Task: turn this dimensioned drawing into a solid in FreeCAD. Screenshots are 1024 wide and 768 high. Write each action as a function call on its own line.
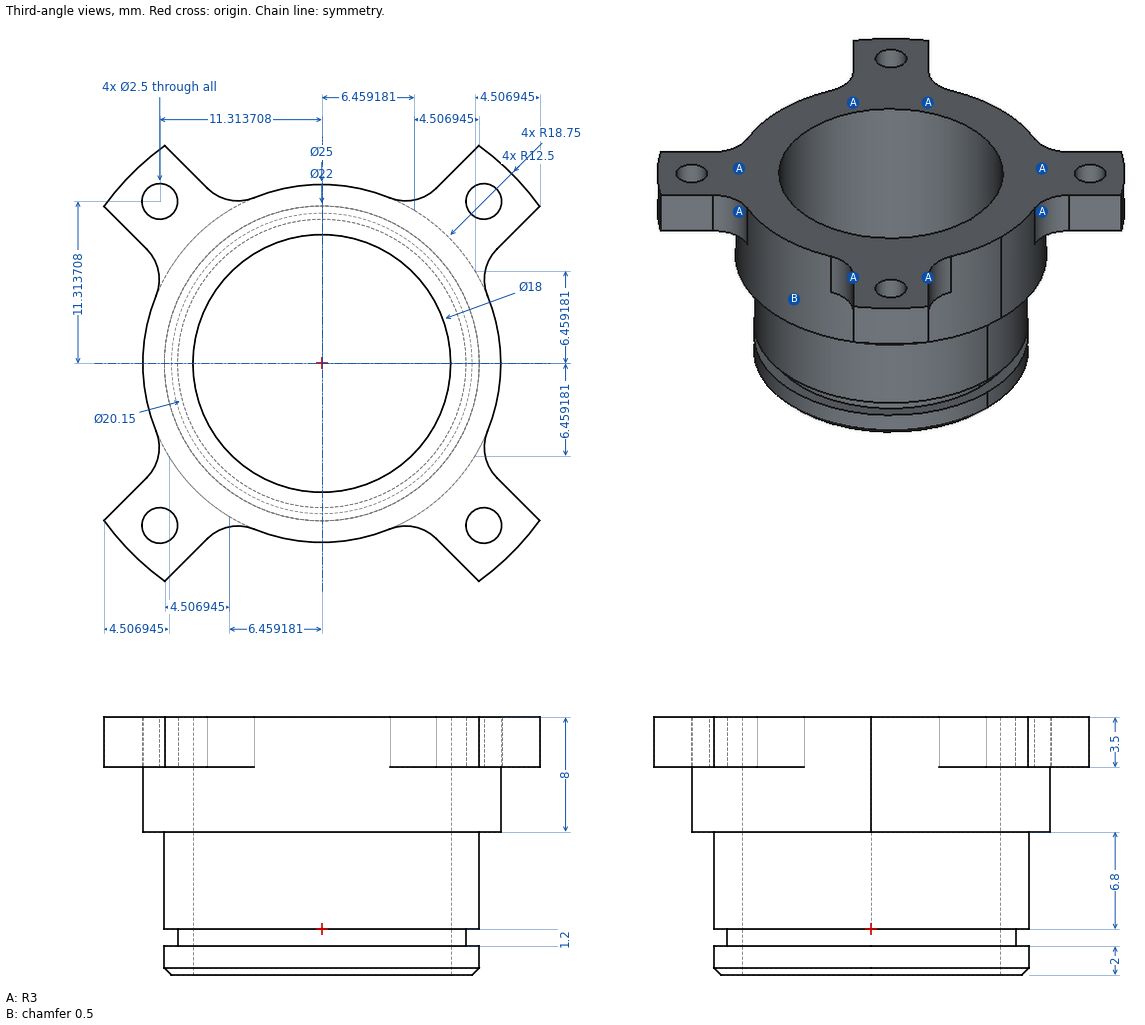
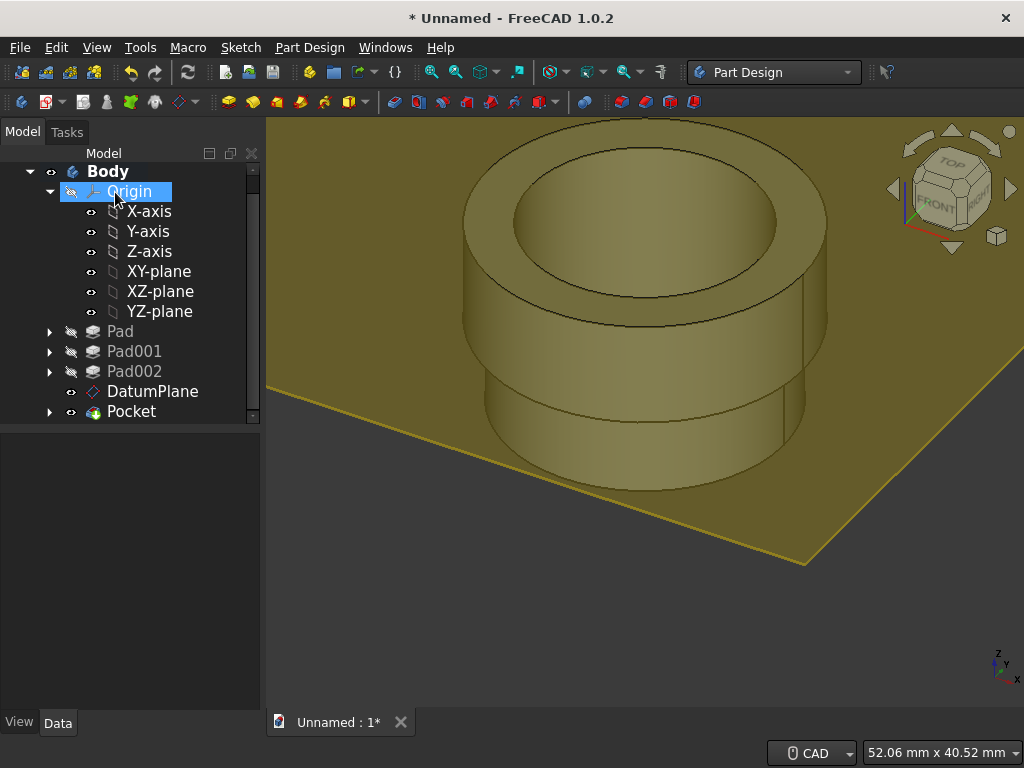
click(116, 392)
key(space)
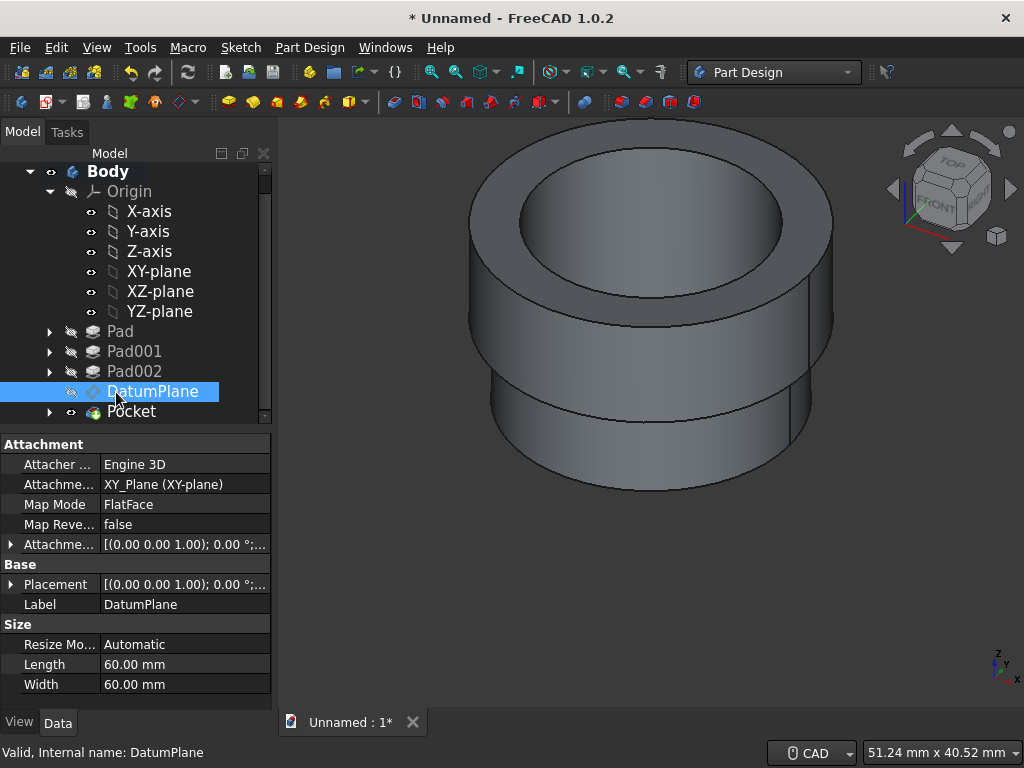
click(432, 72)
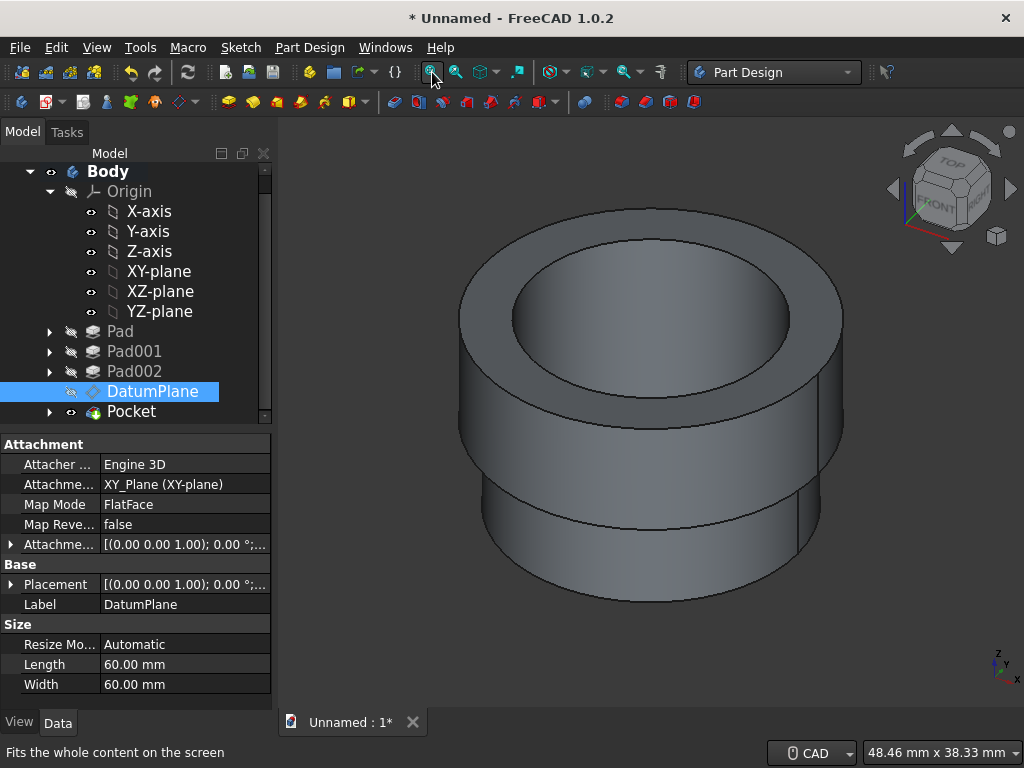
click(136, 272)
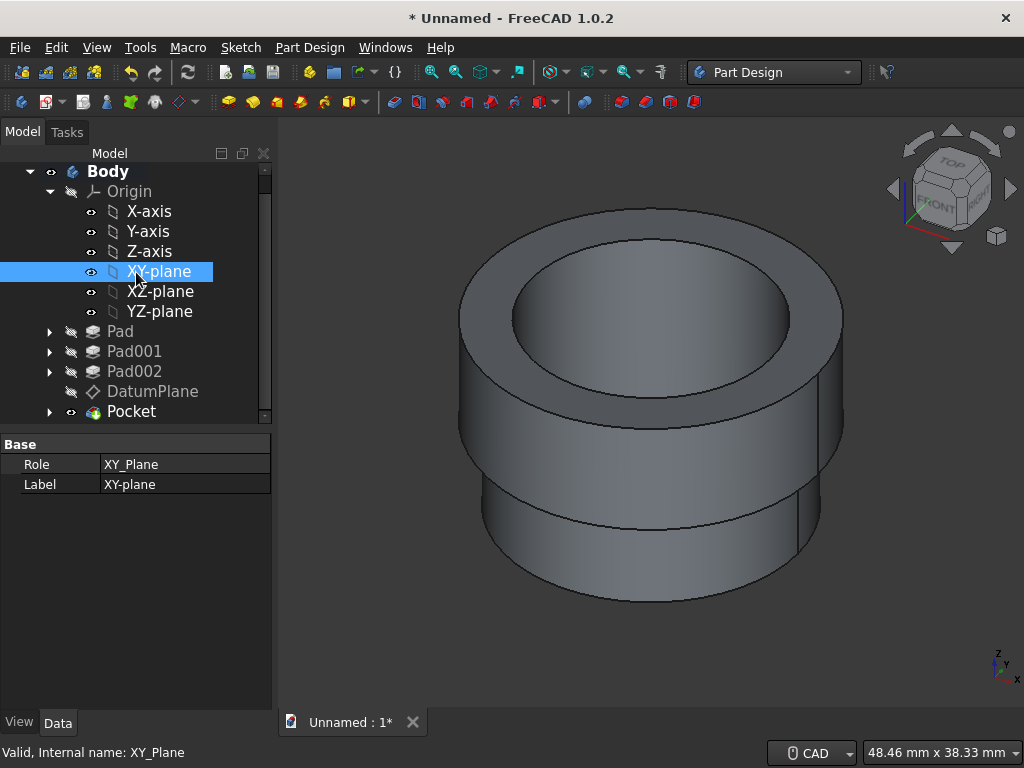
click(180, 102)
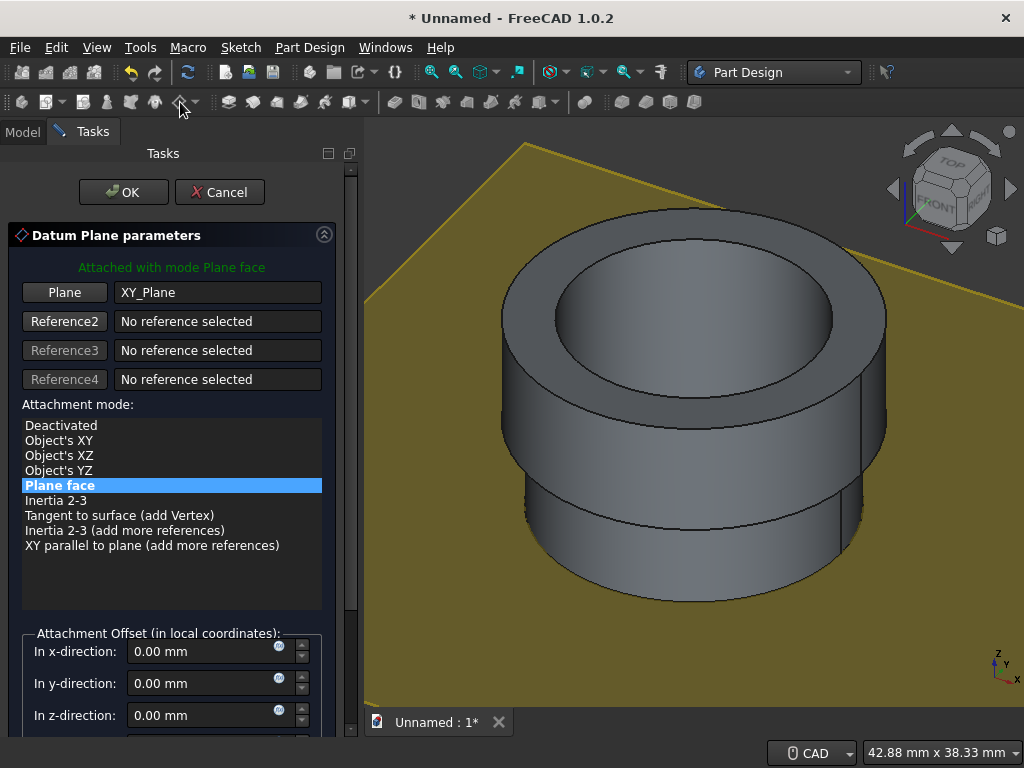
triple_click(210, 715)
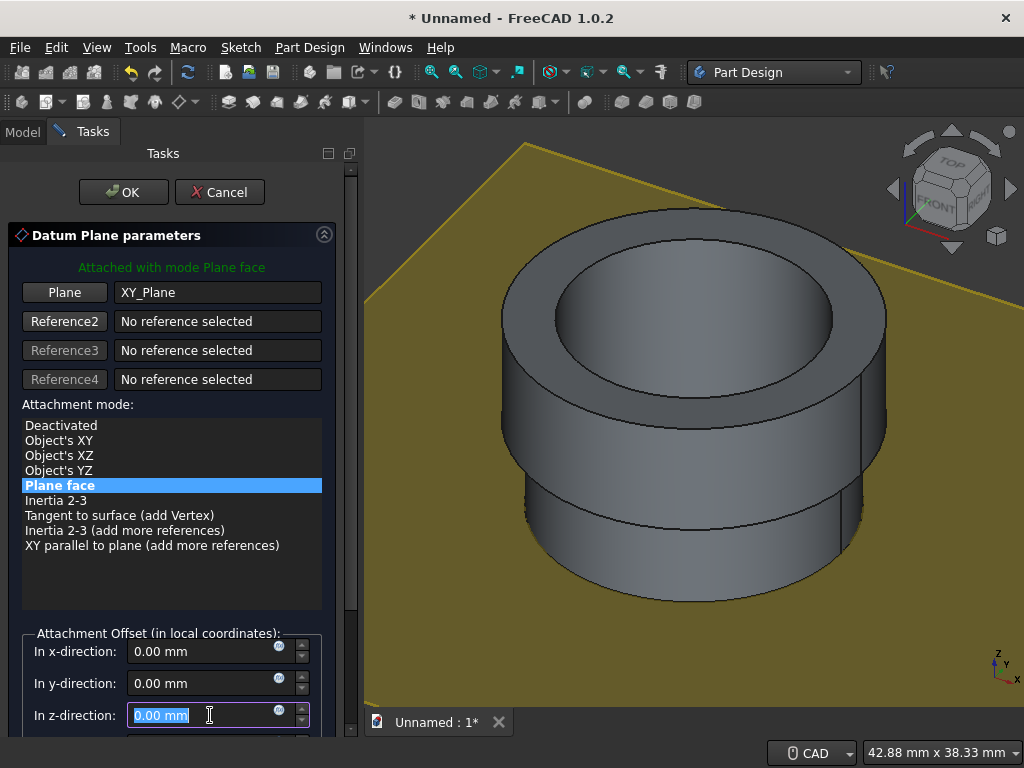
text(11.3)
key(Tab)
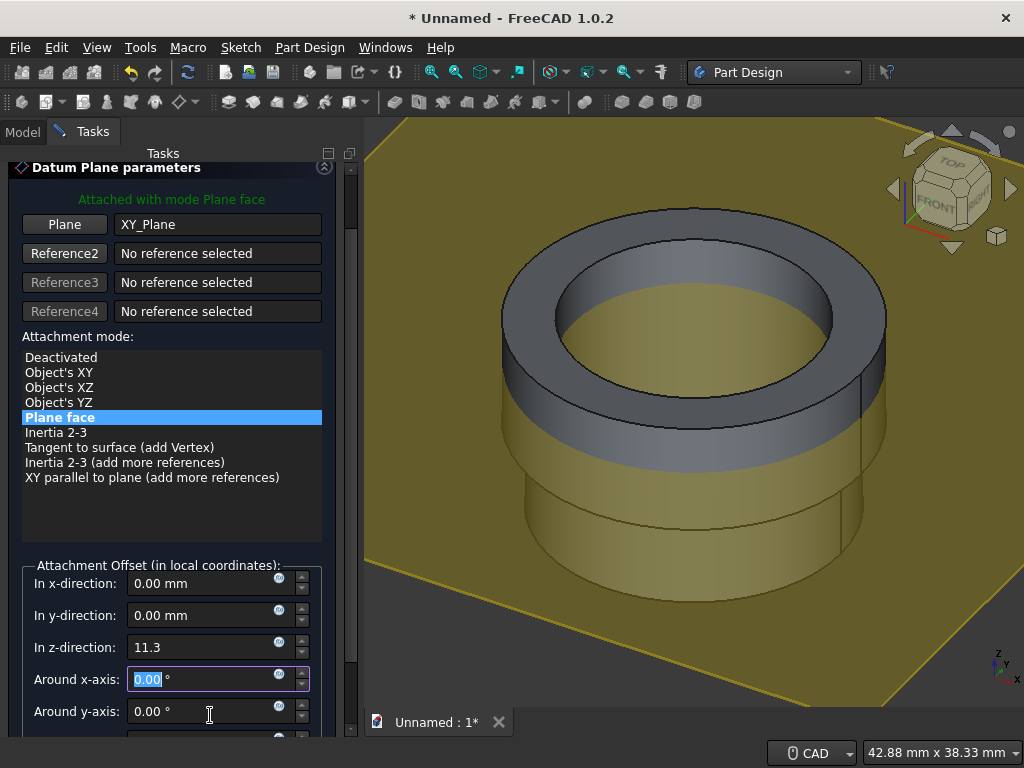
scroll(351, 450, up, 2)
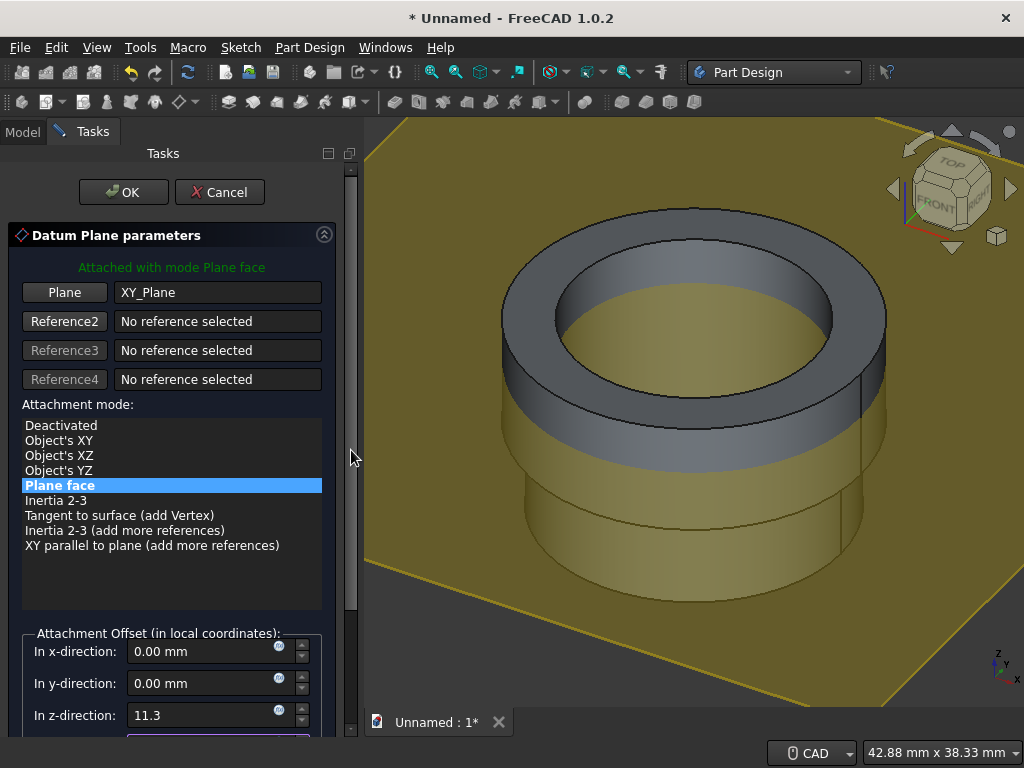
click(124, 192)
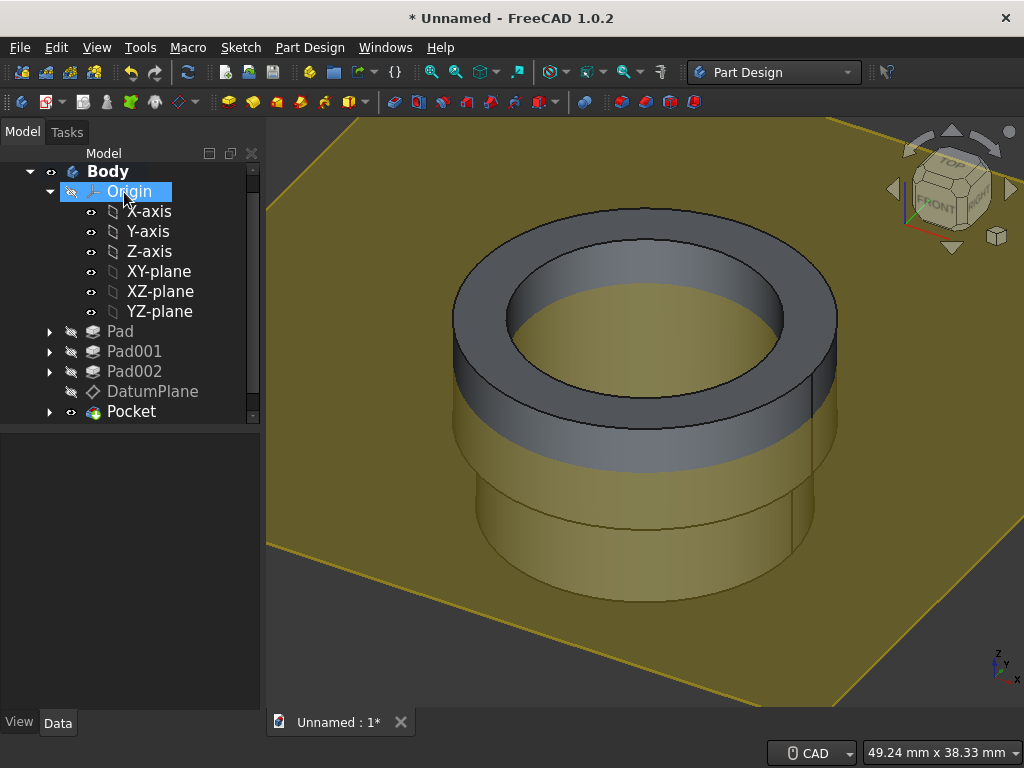
scroll(120, 287, down, 3)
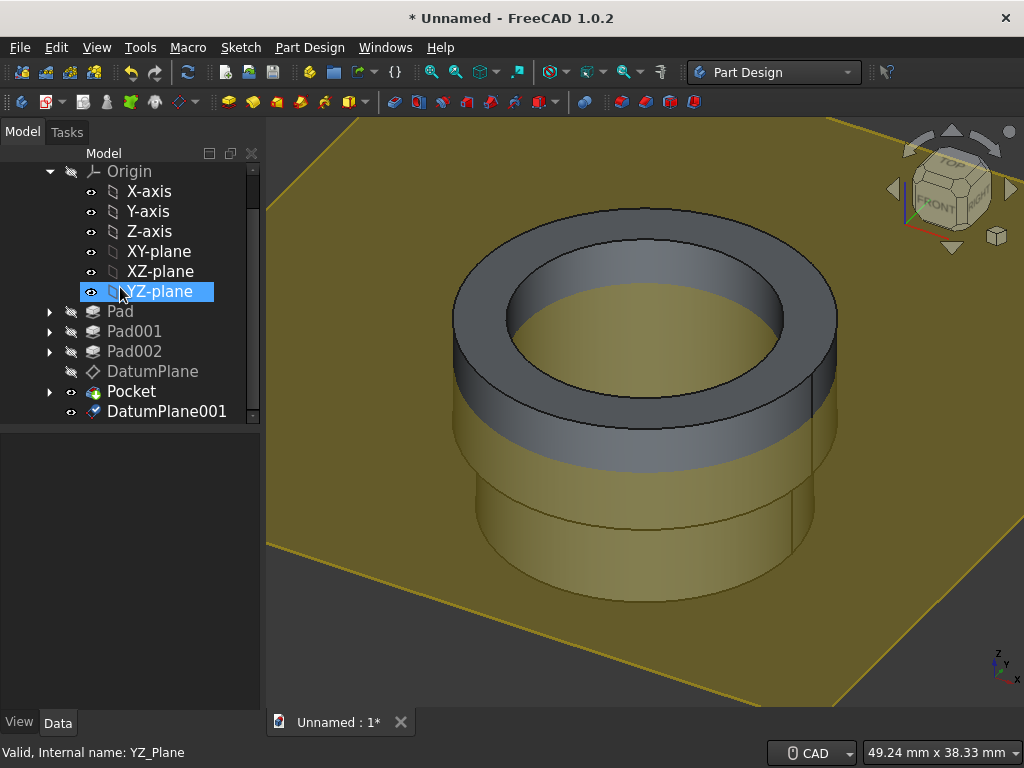
click(116, 412)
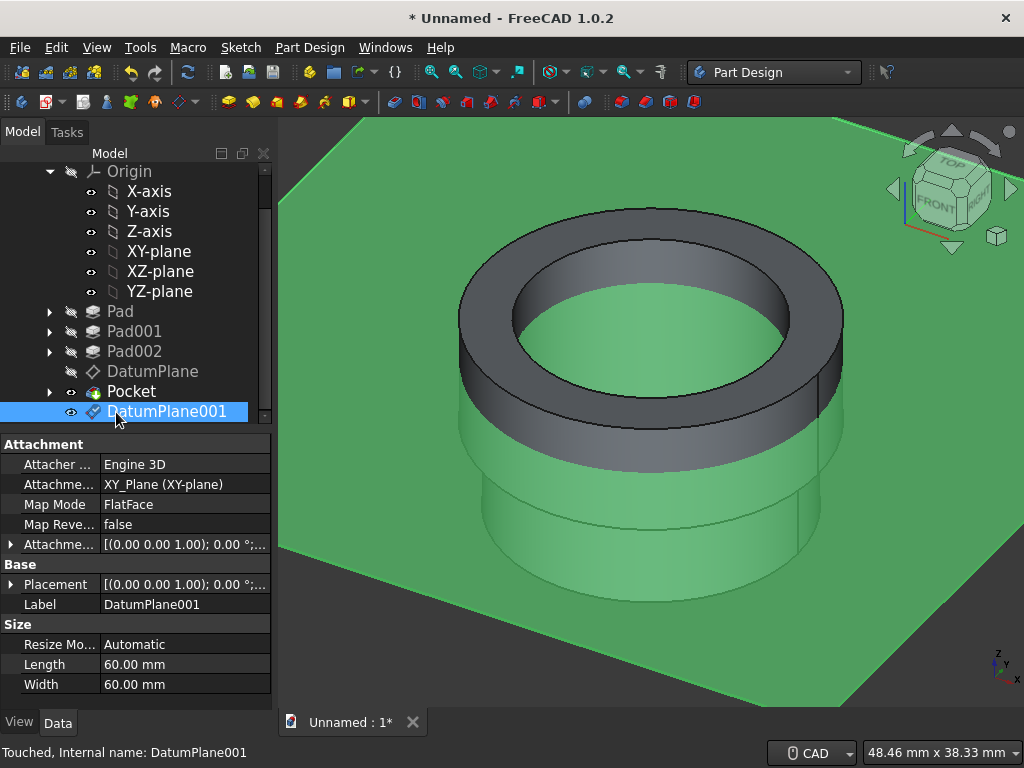
click(46, 102)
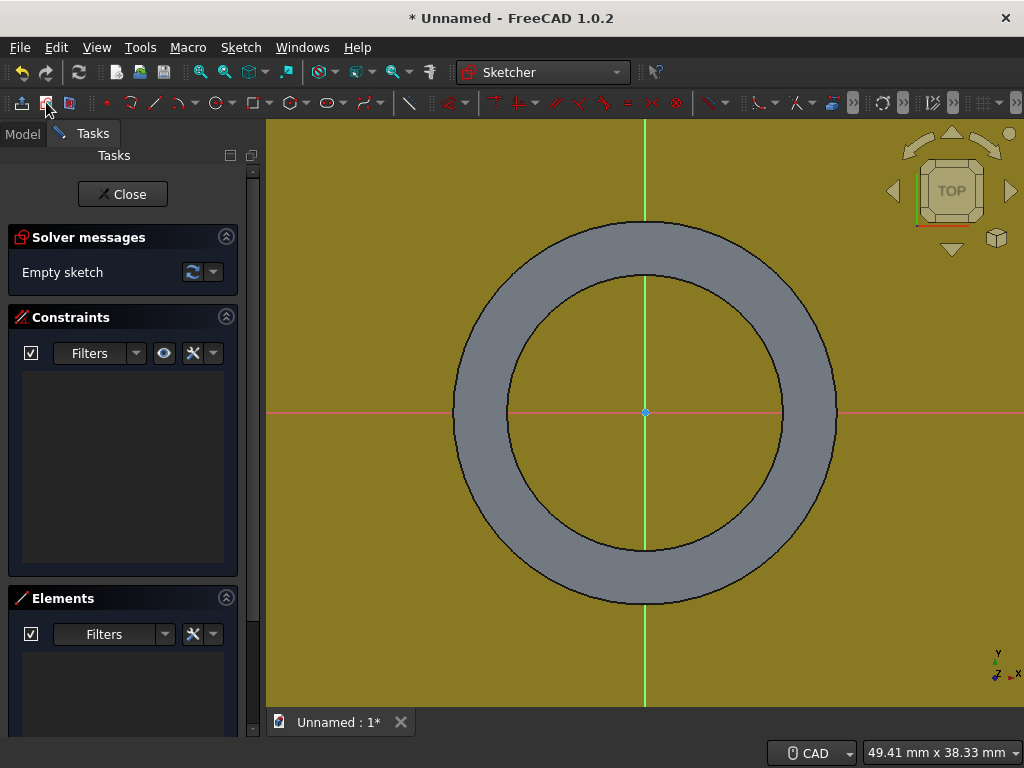
click(70, 104)